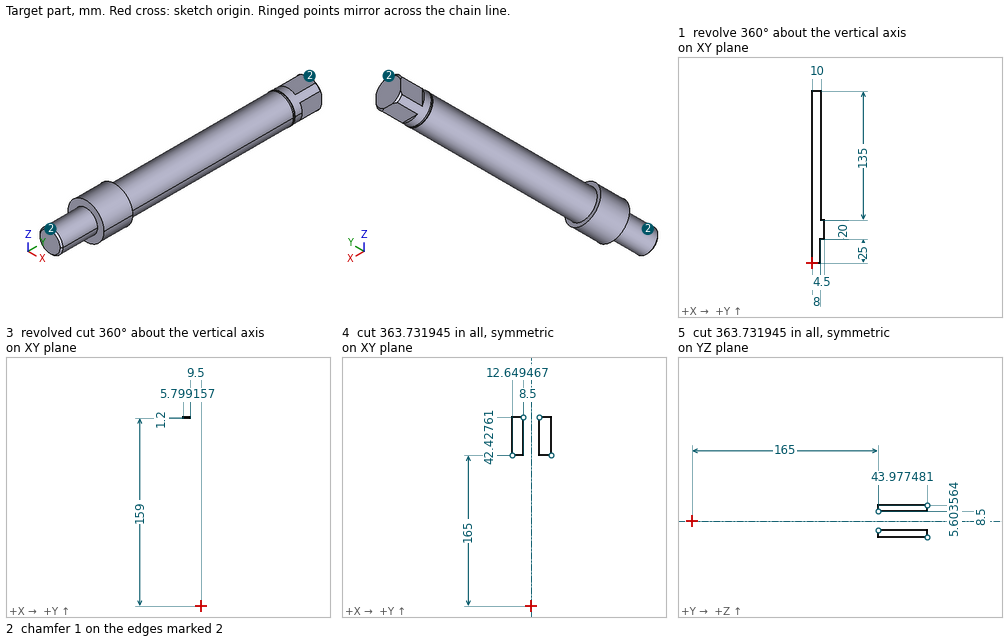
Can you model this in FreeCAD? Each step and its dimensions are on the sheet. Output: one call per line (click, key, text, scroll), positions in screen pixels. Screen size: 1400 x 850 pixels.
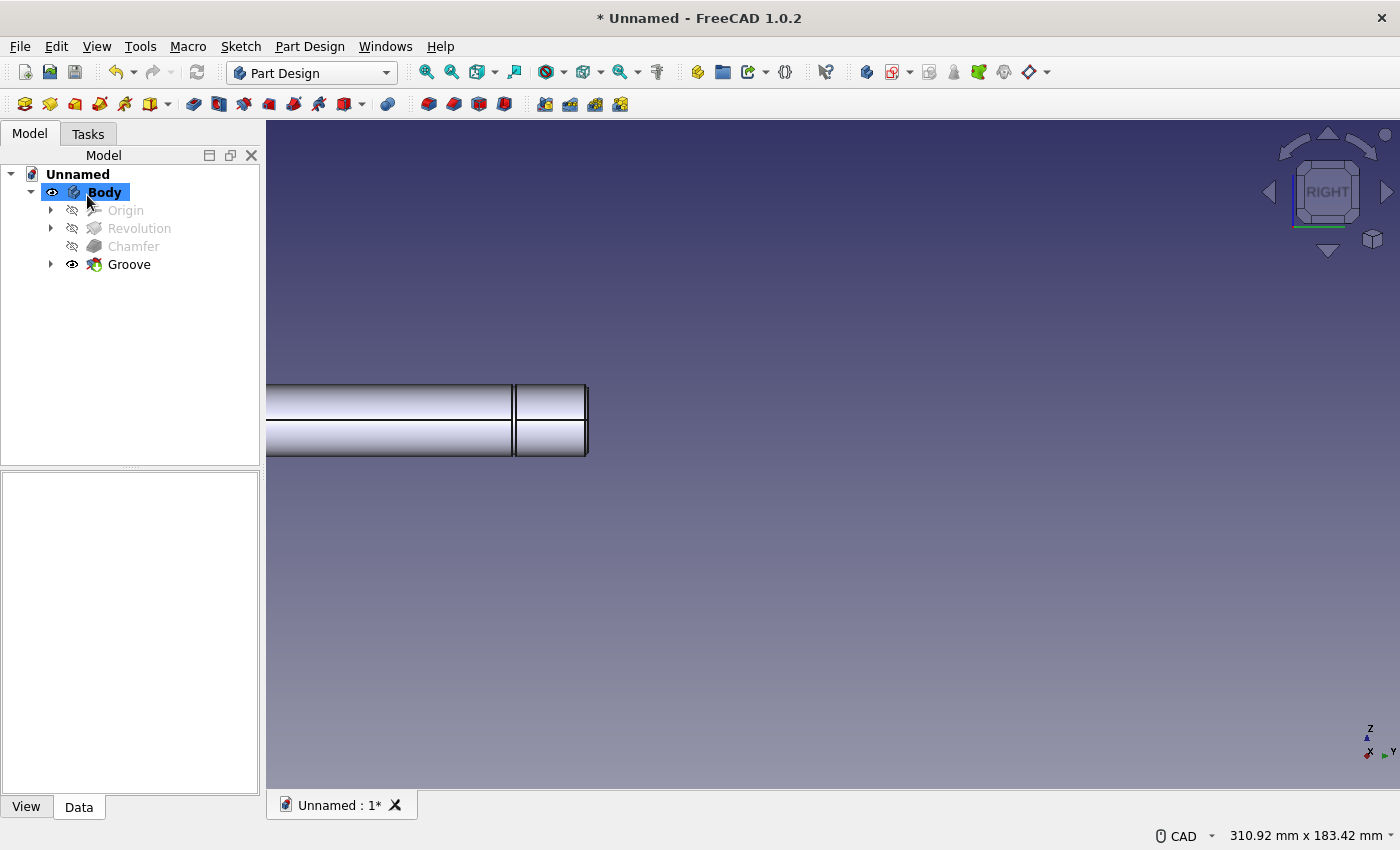
key(v)
key(f)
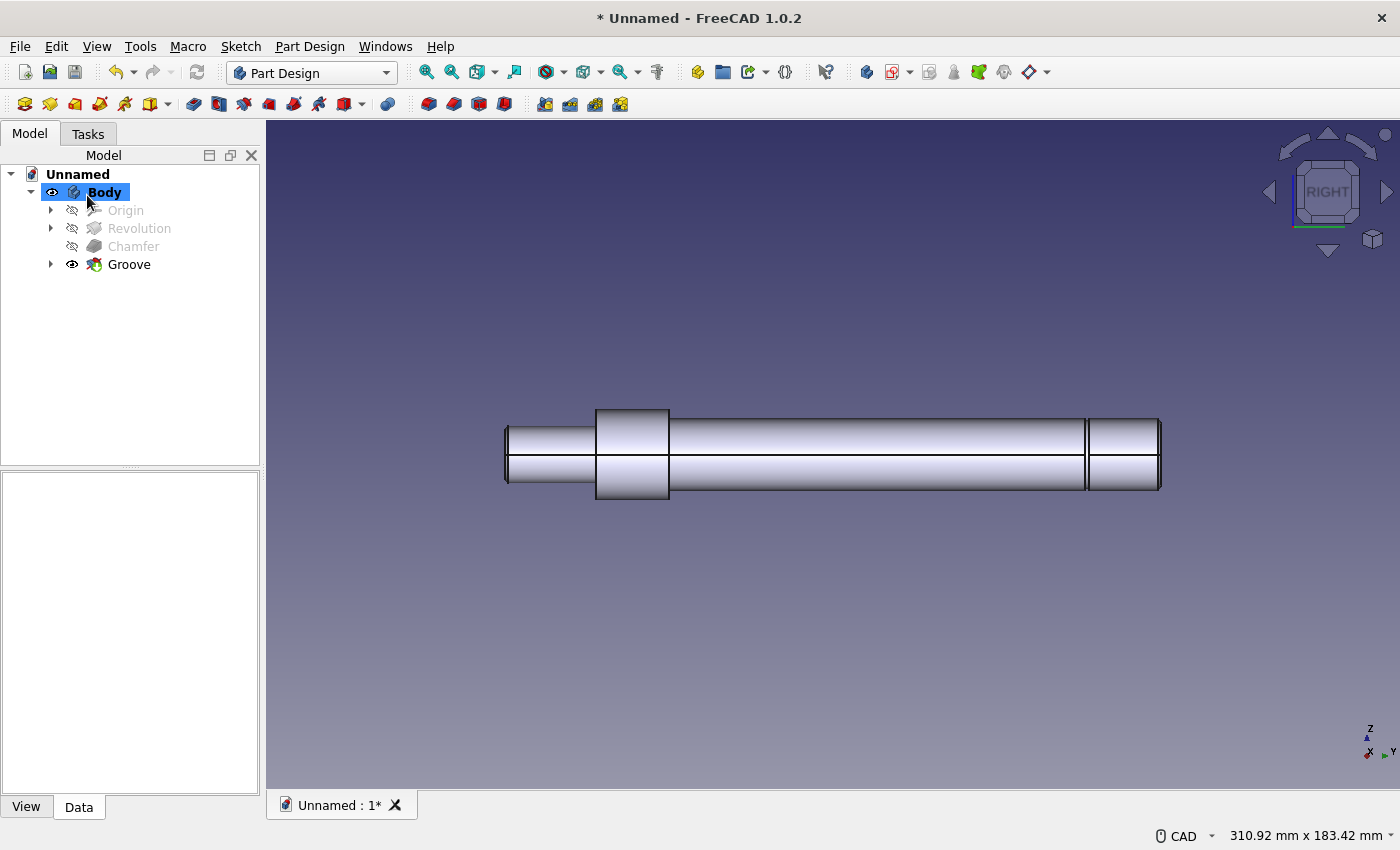
click(892, 72)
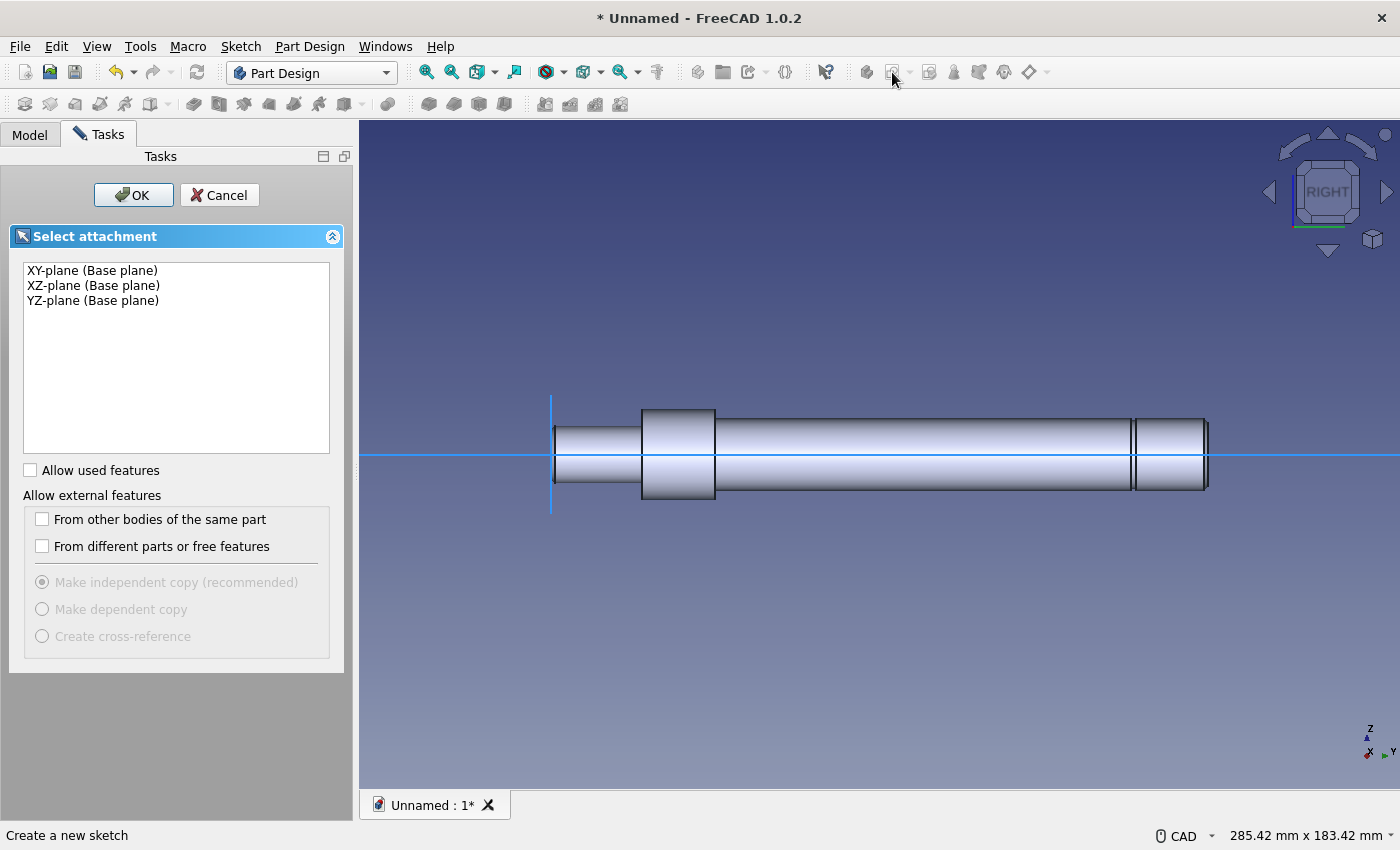
click(84, 270)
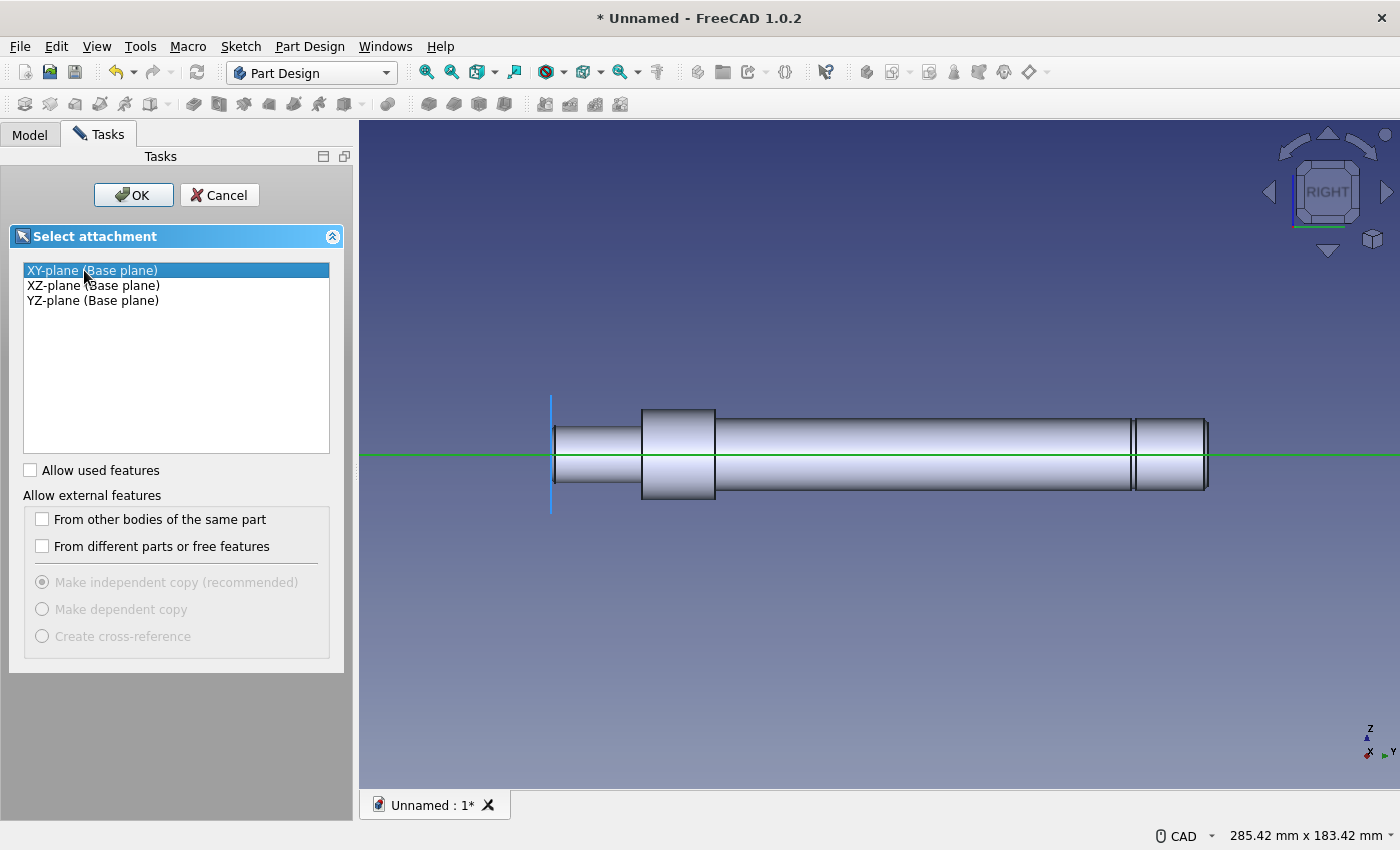
click(134, 195)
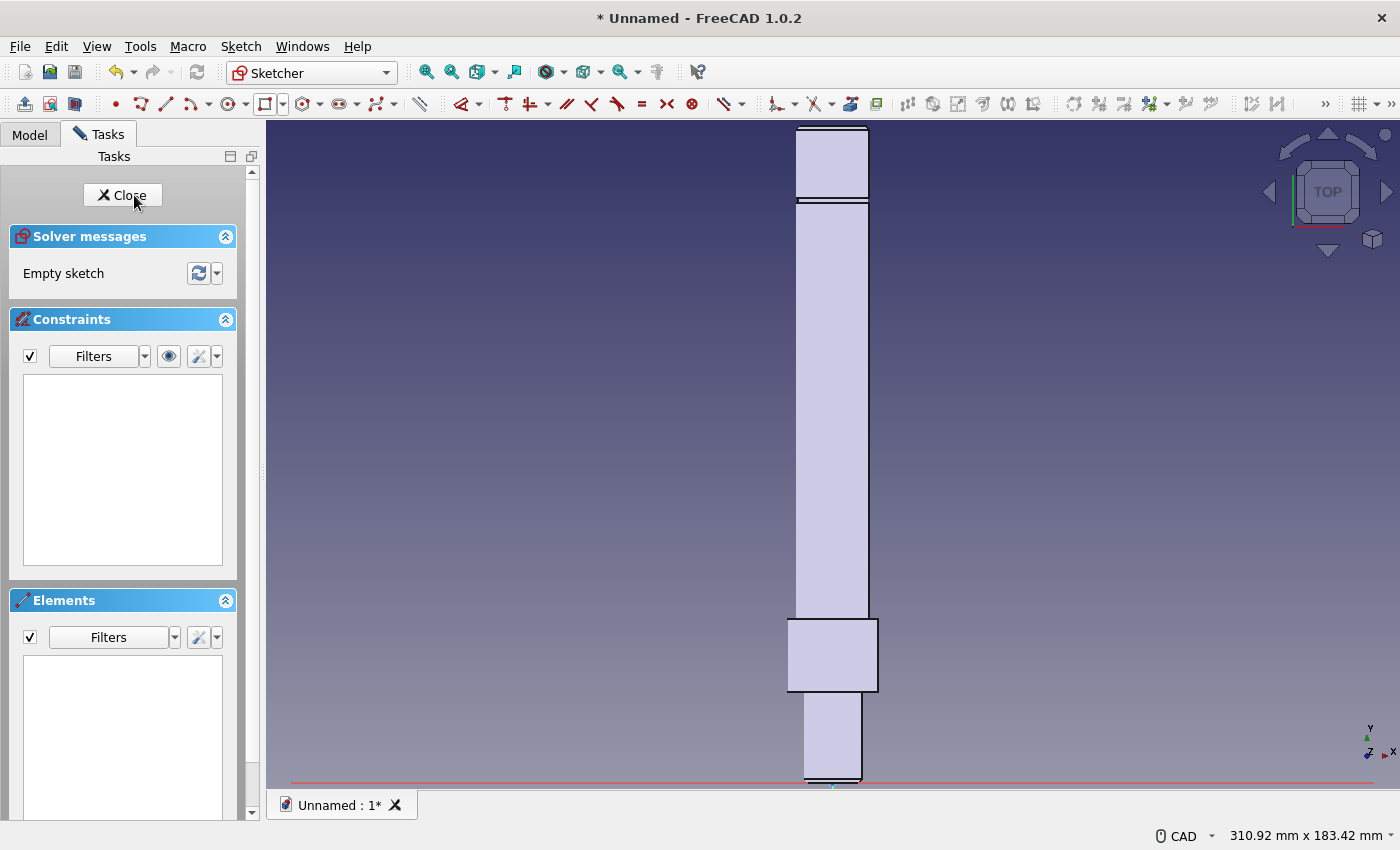
click(75, 104)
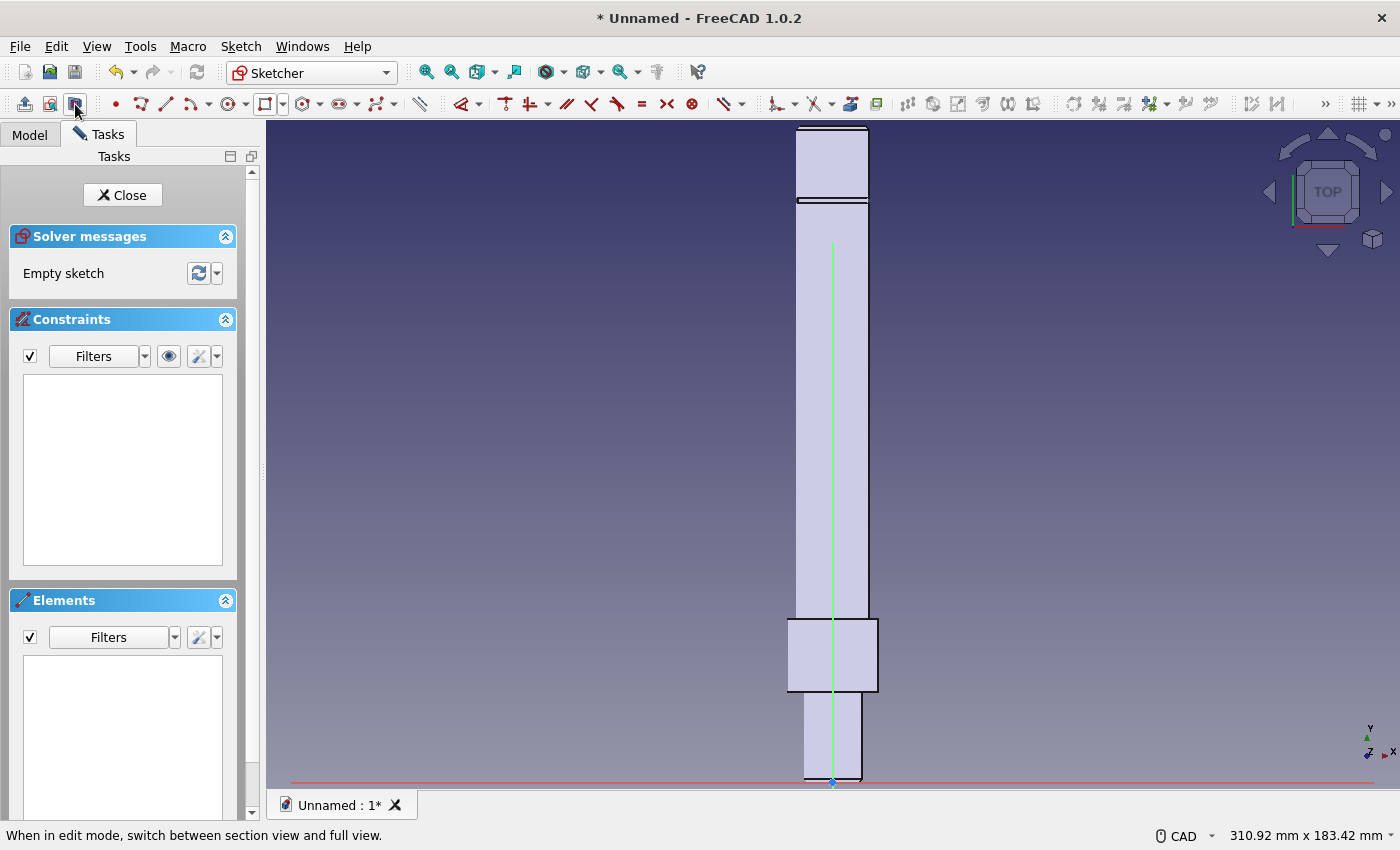
scroll(764, 454, down, 5)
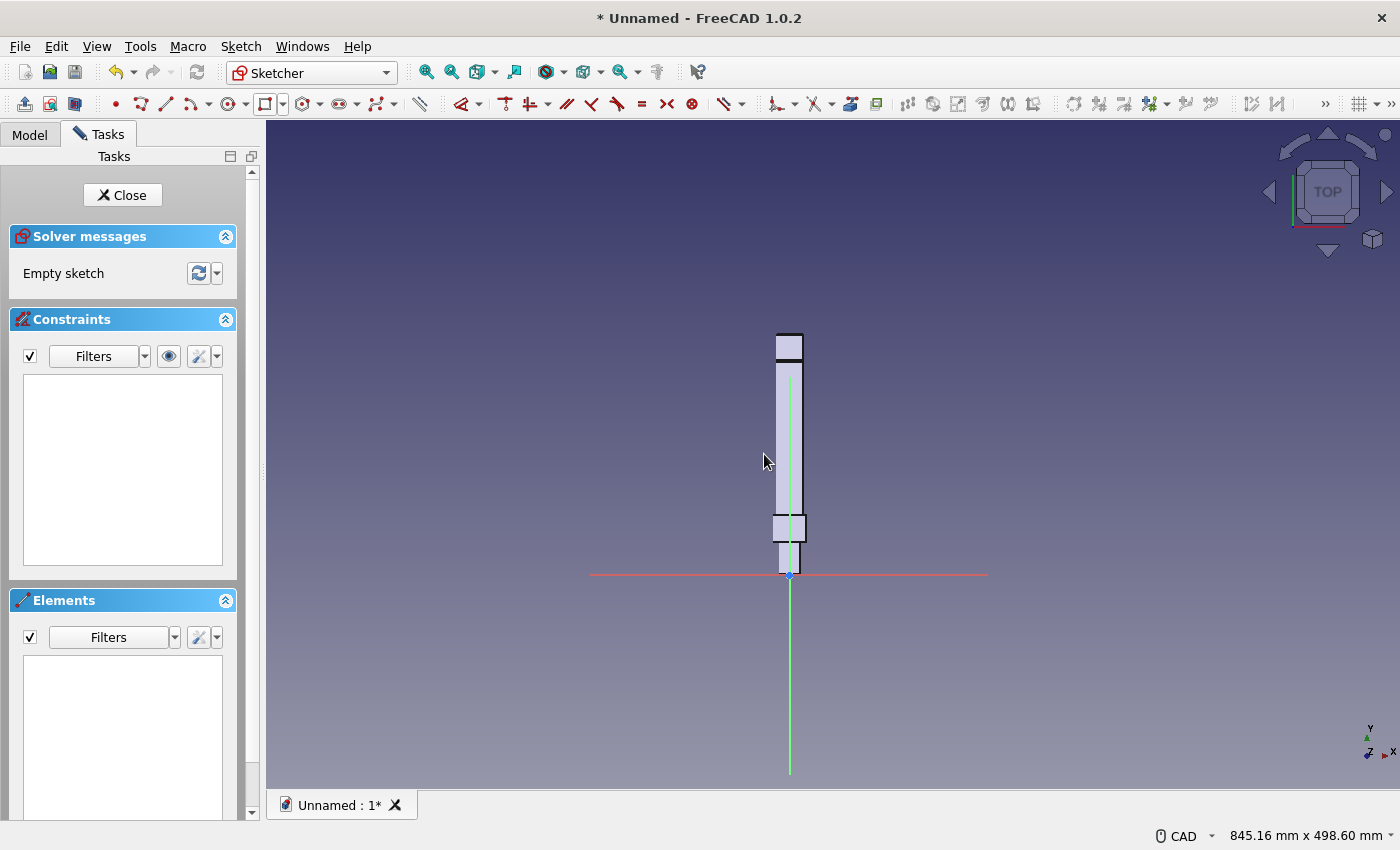
scroll(794, 305, up, 10)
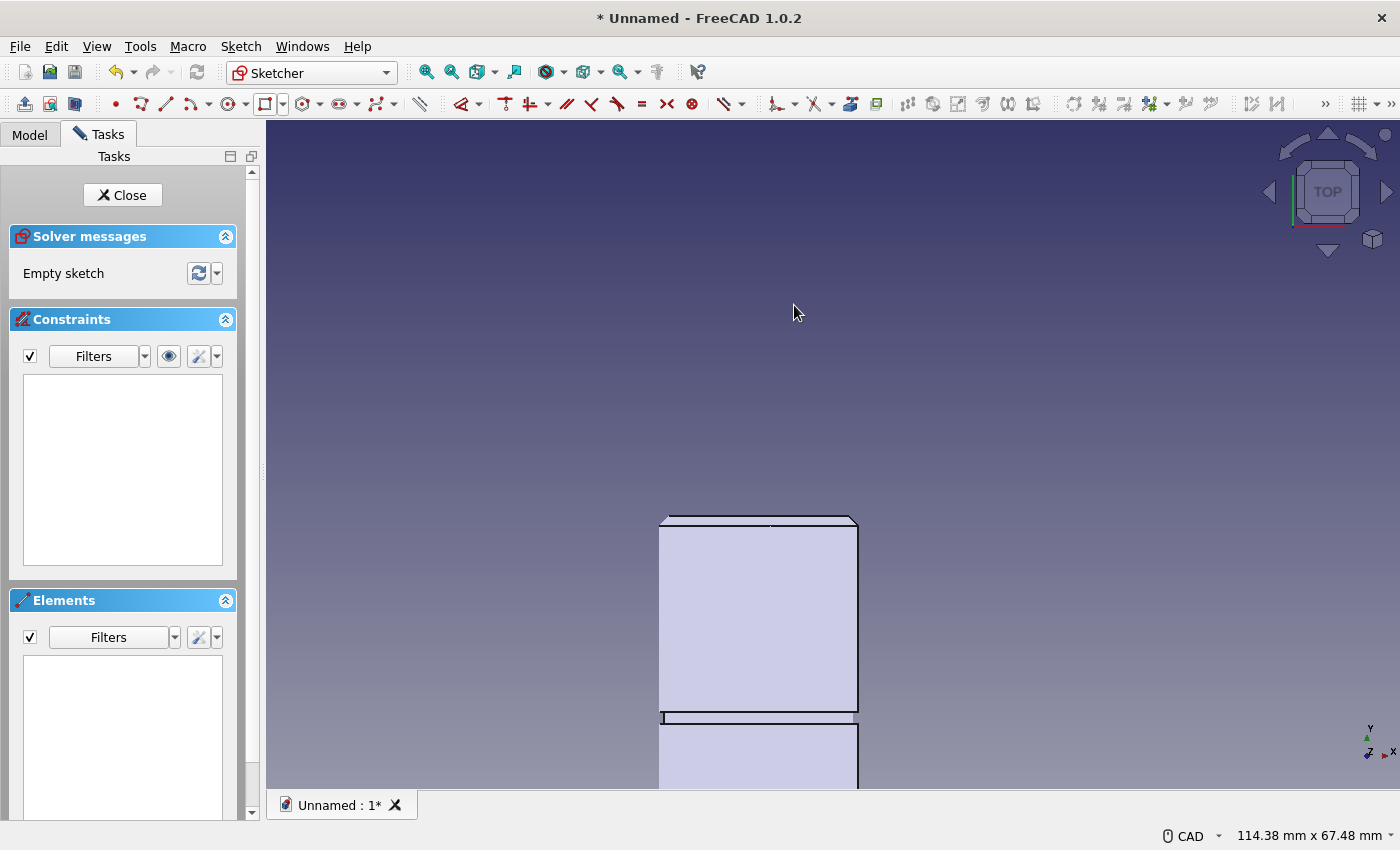
key(g)
key(r)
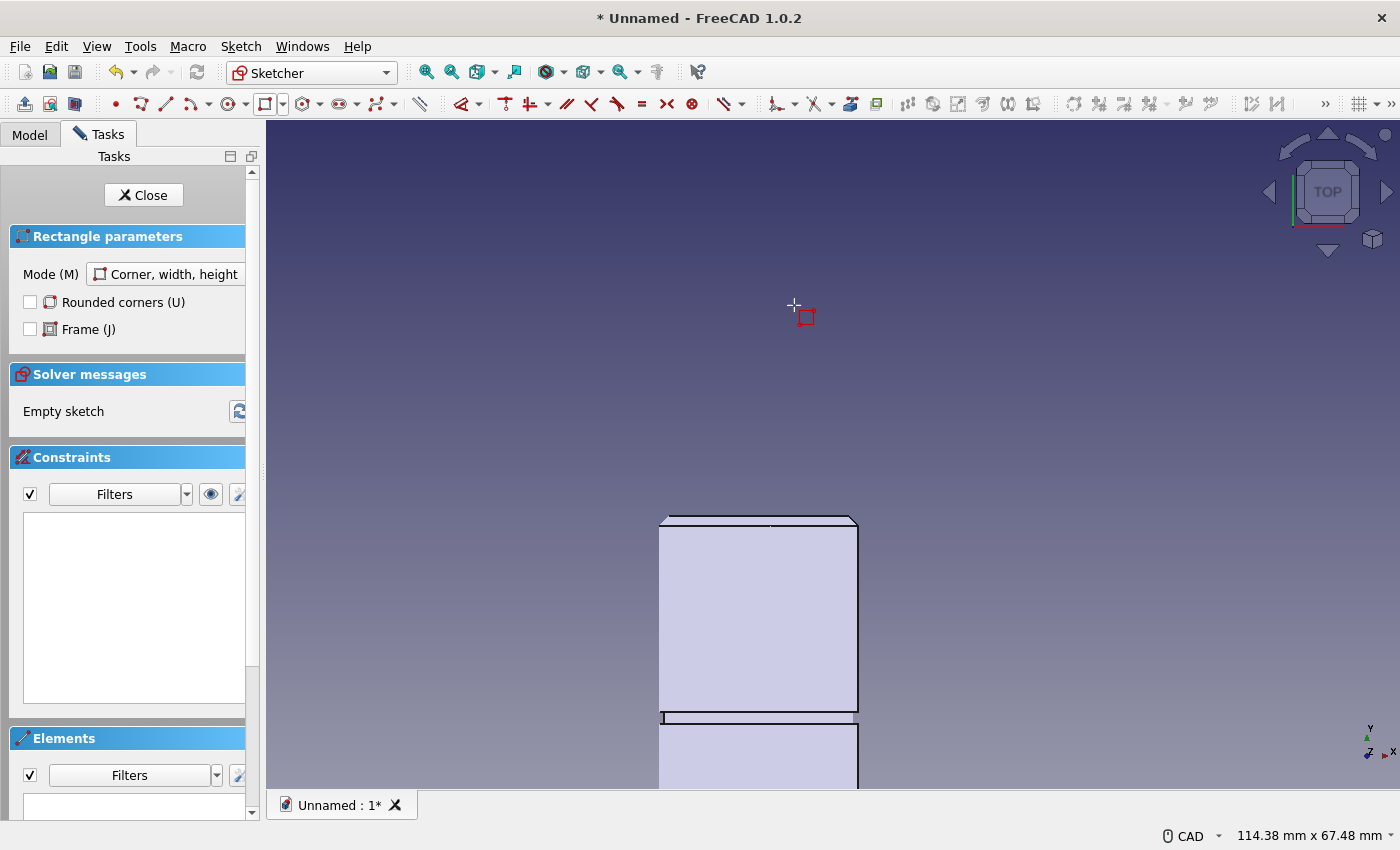
click(549, 244)
click(674, 664)